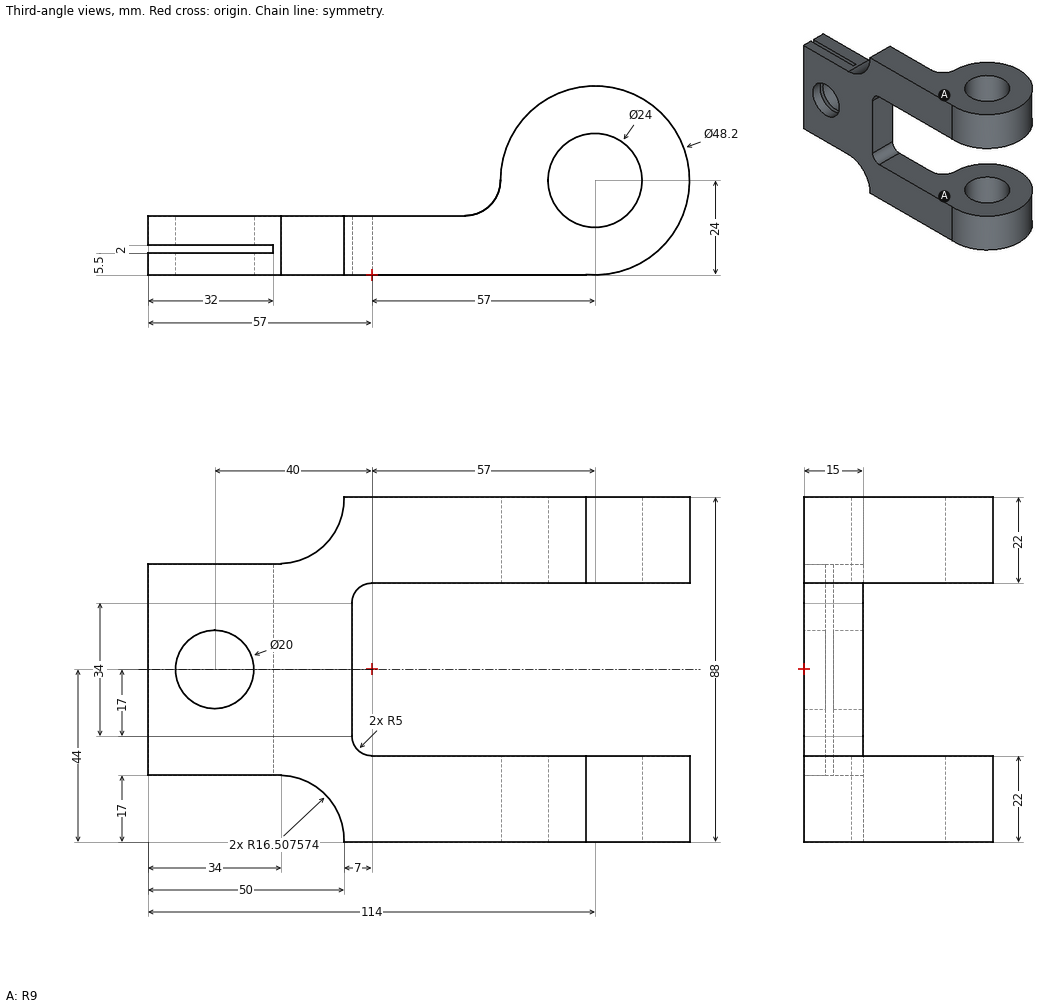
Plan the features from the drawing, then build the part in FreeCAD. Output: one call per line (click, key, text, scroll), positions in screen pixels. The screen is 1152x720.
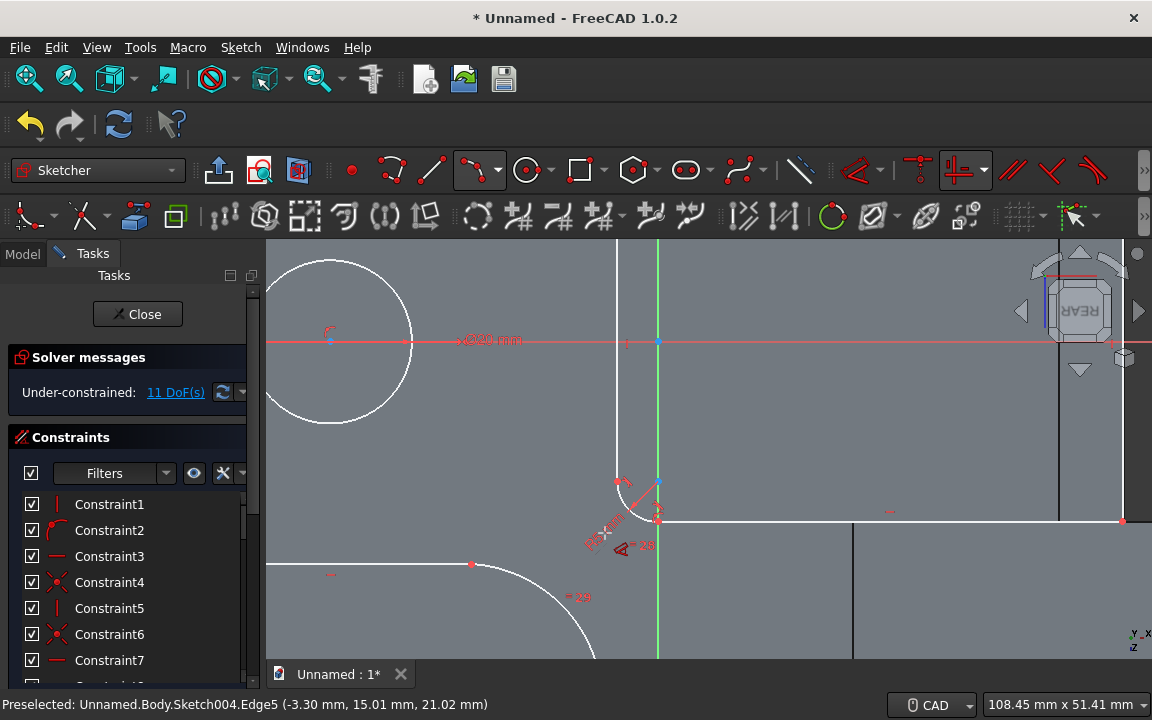
scroll(630, 511, down, 5)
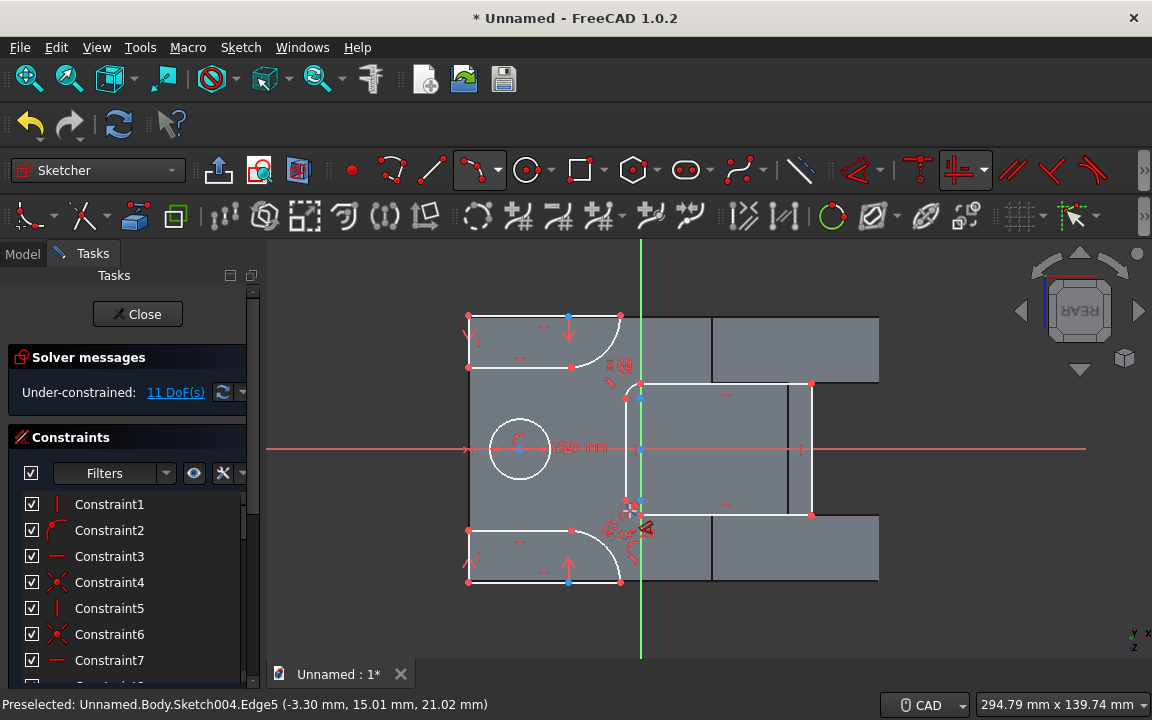
click(594, 361)
click(610, 389)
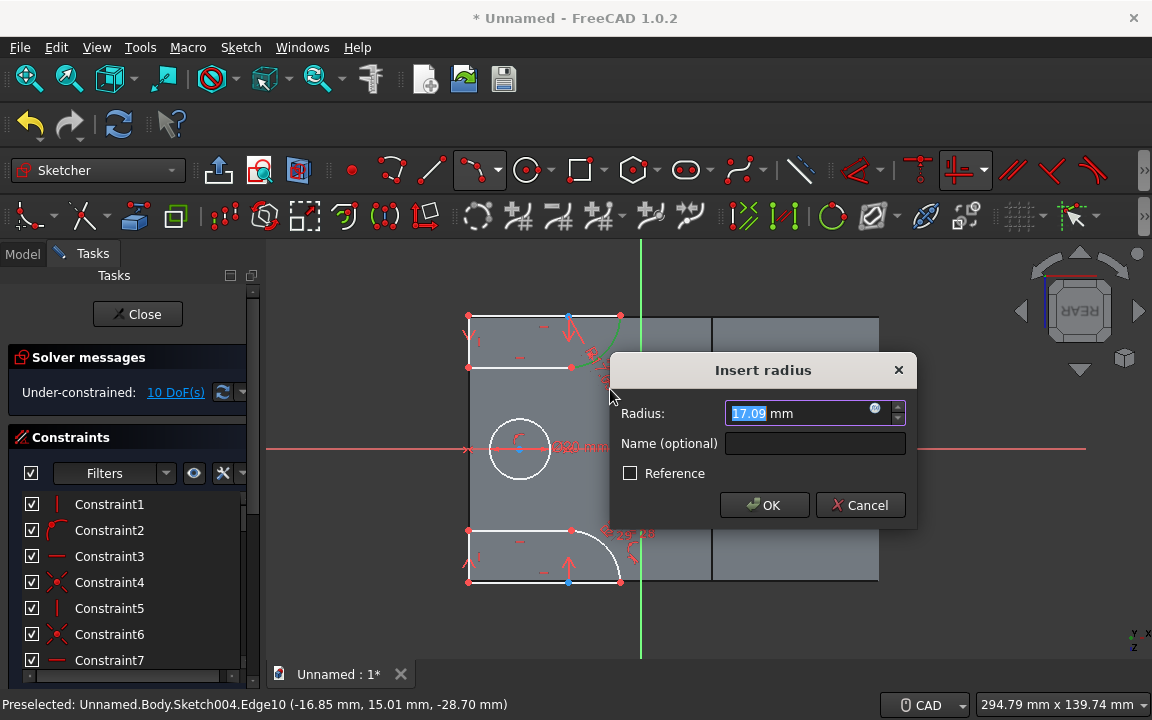
text(16.507574)
key(Return)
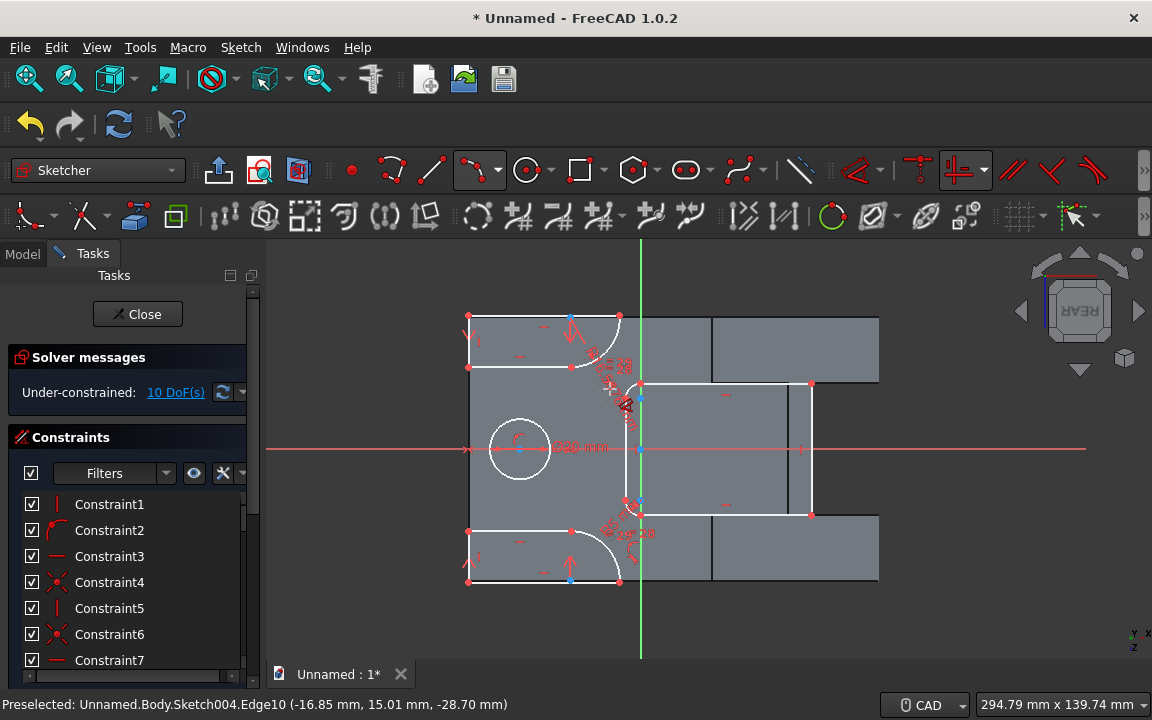
click(626, 429)
click(592, 426)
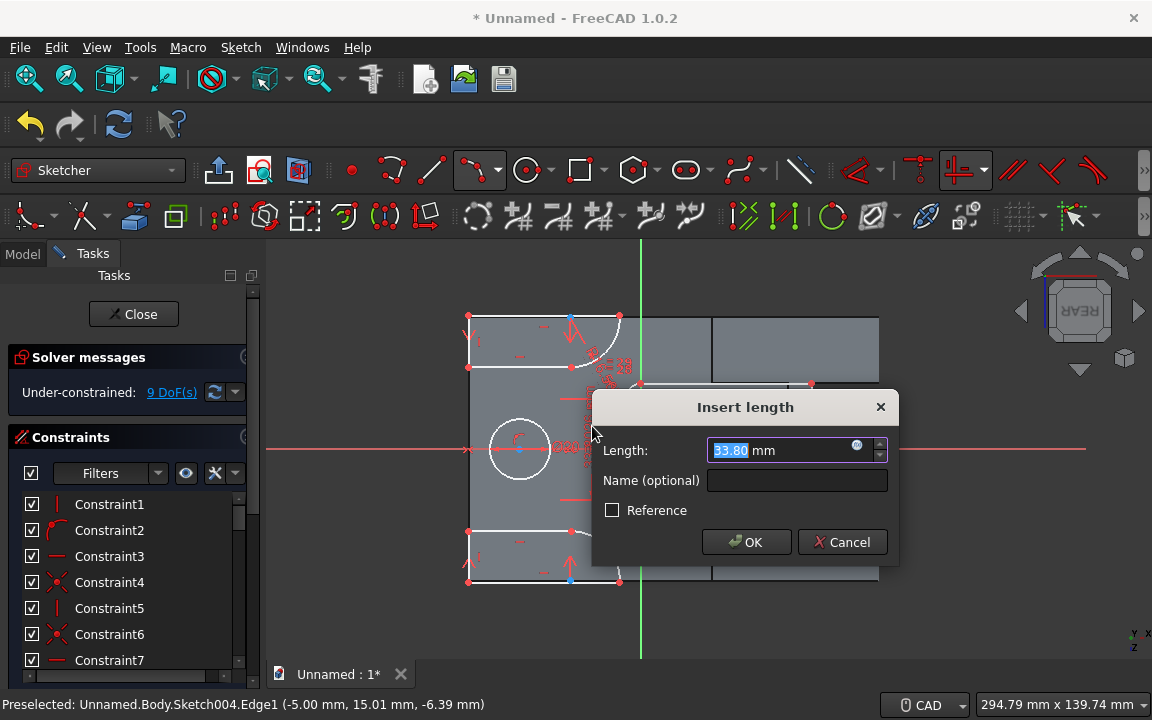
text(34)
key(Return)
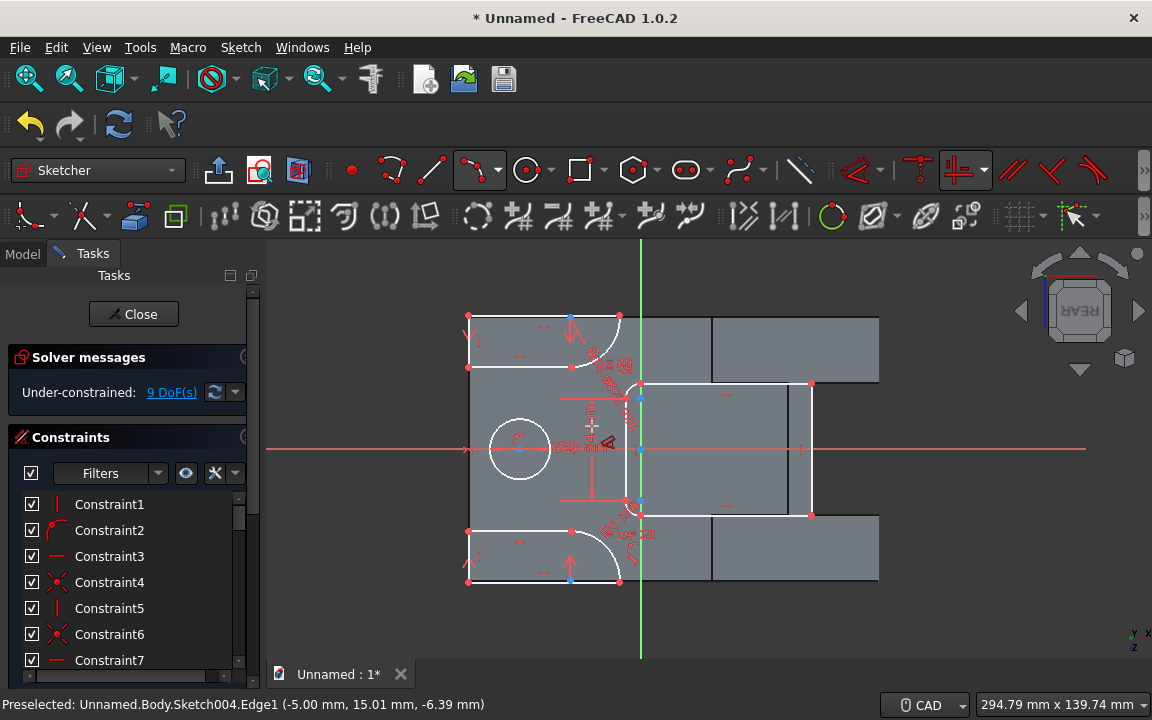
click(692, 516)
click(726, 550)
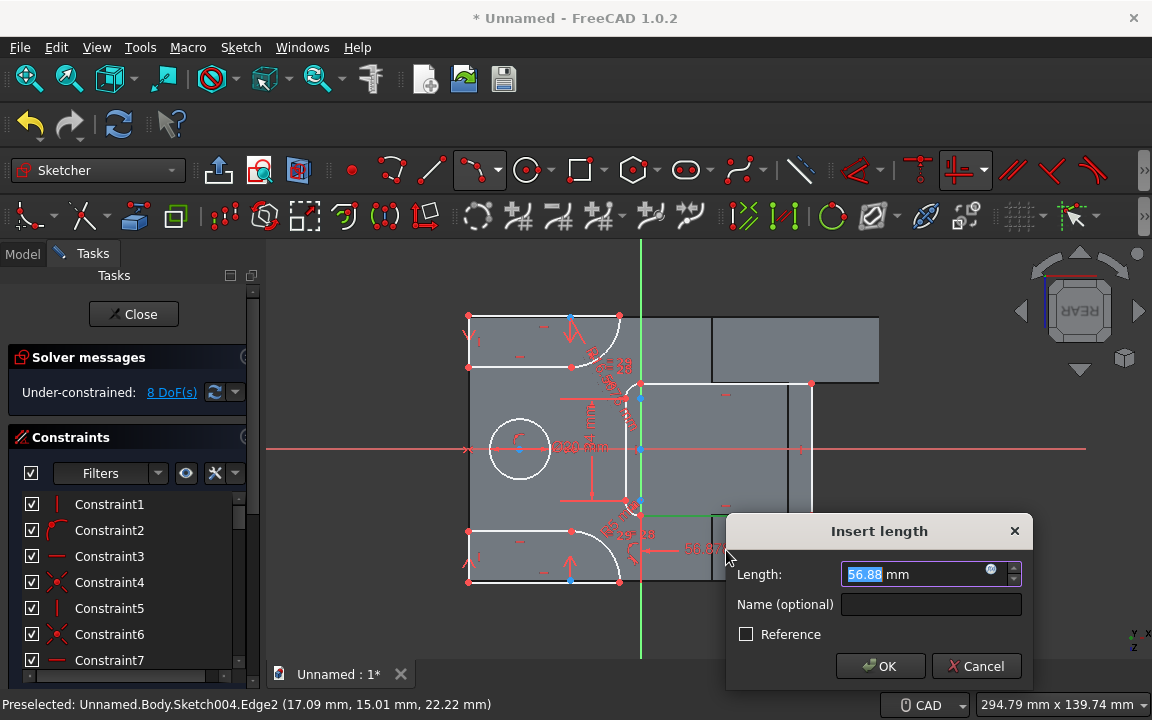
text(57)
key(Return)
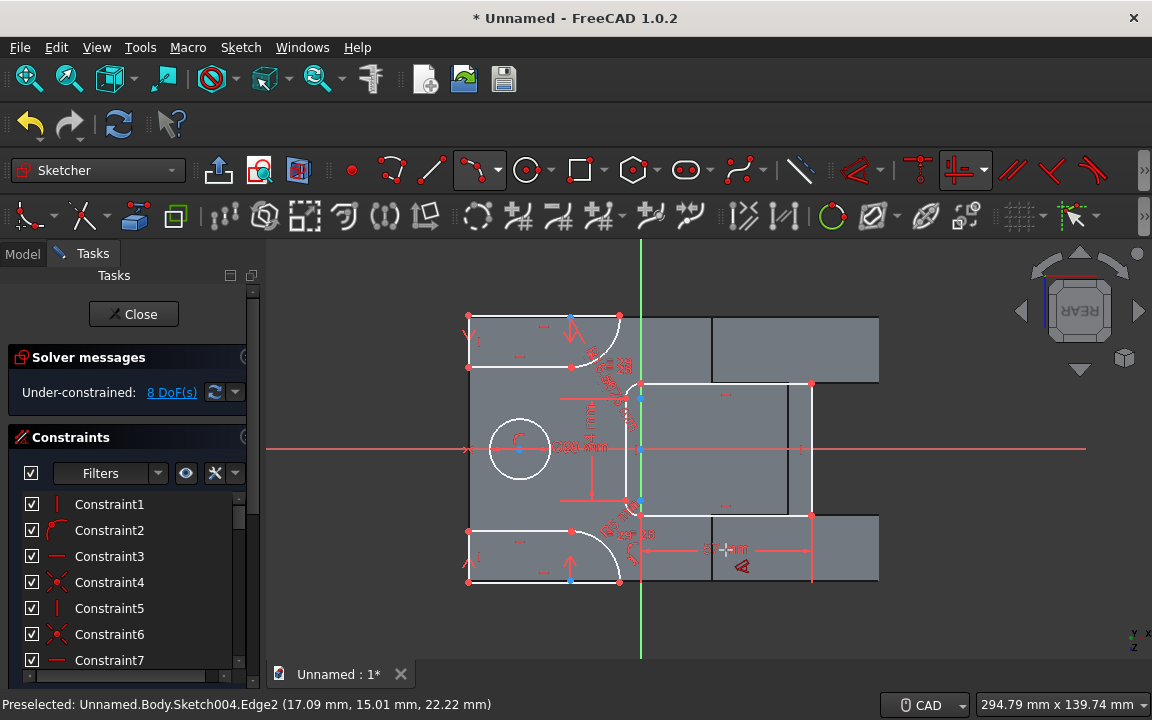
click(514, 316)
click(544, 282)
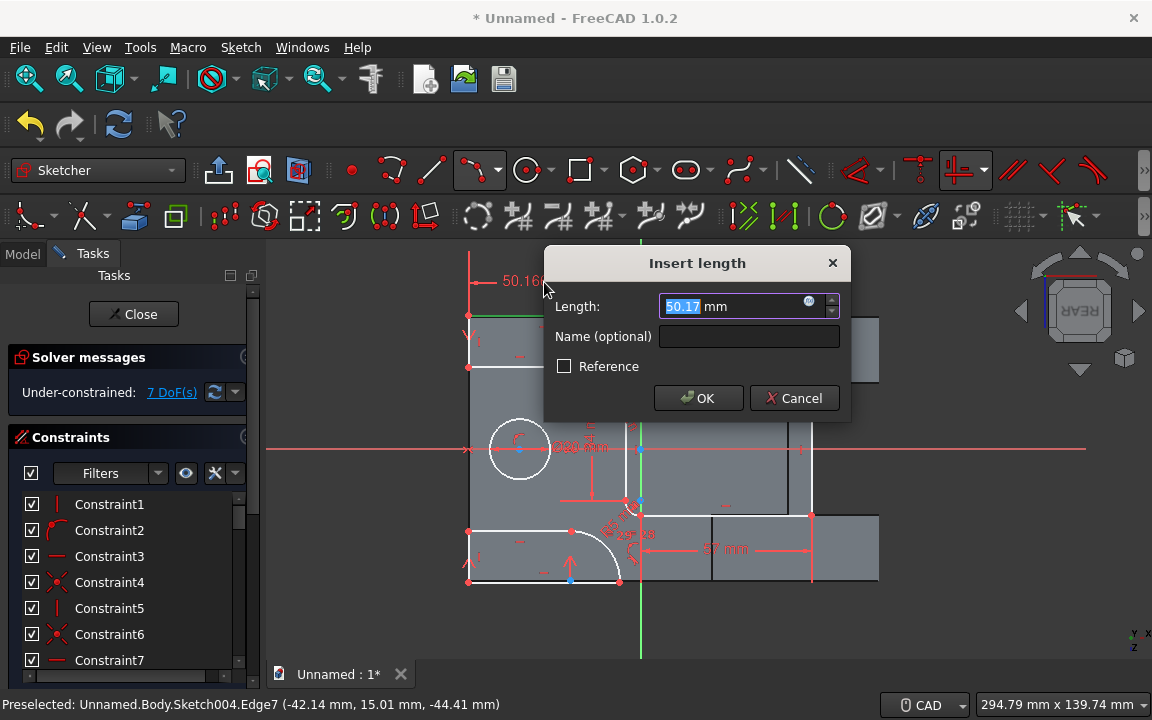
text(50)
key(Return)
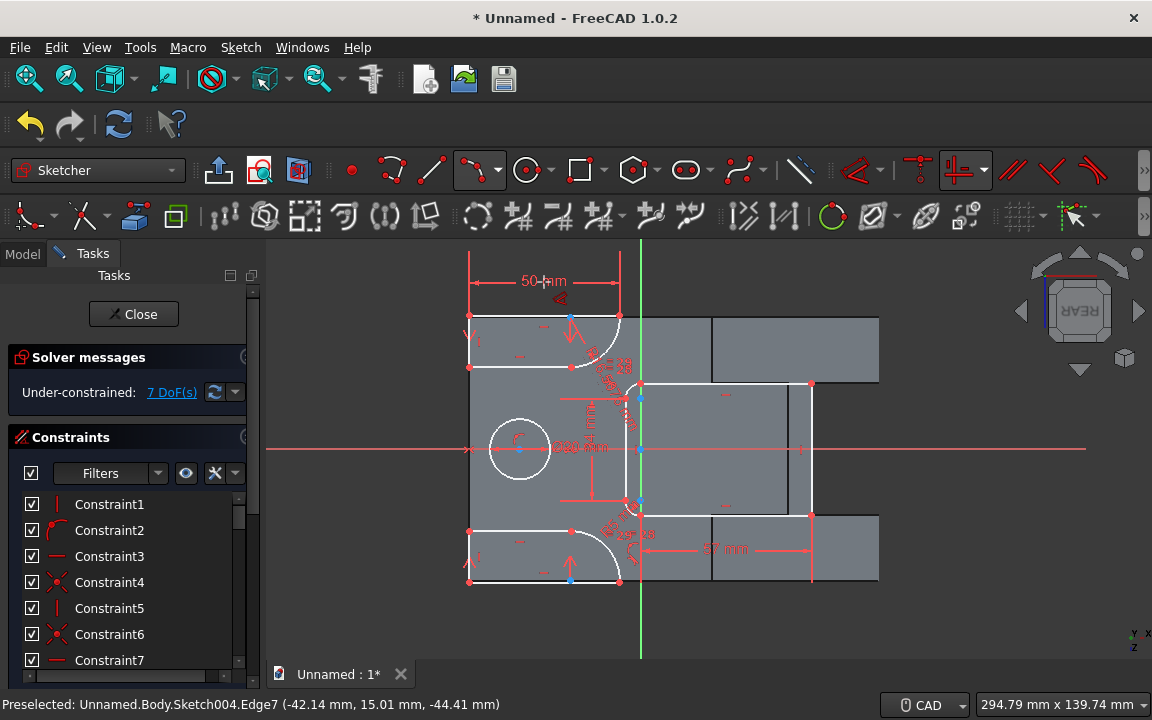
click(469, 331)
click(435, 342)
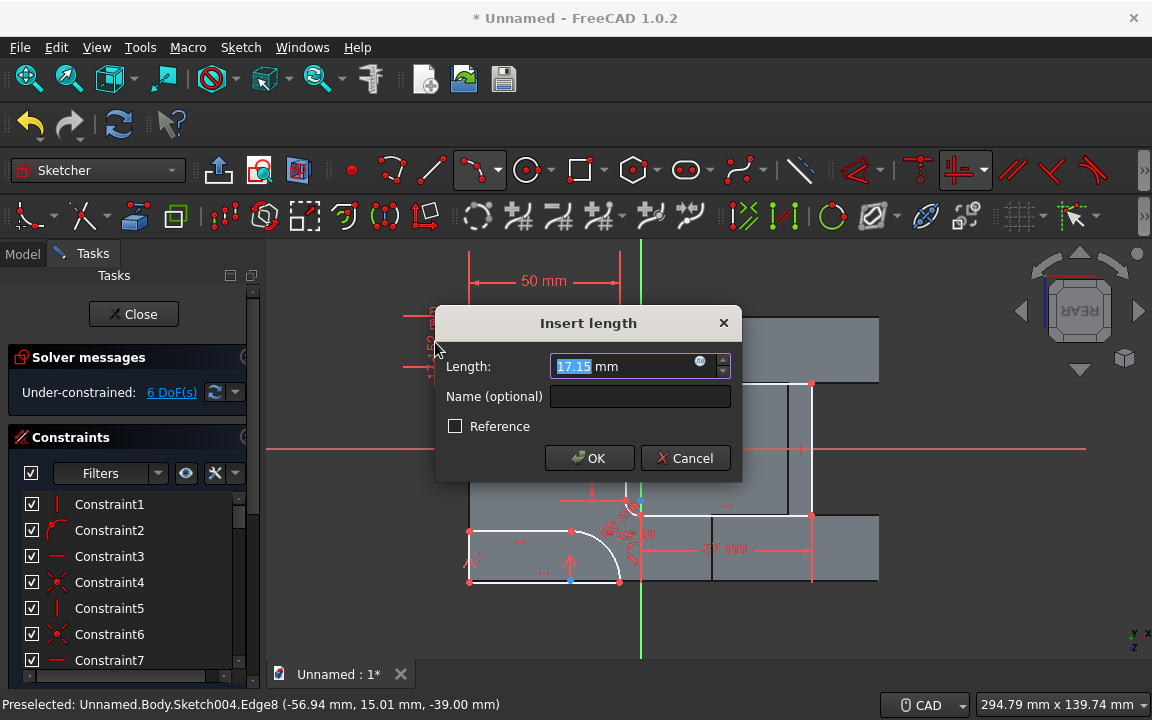
text(17)
key(Return)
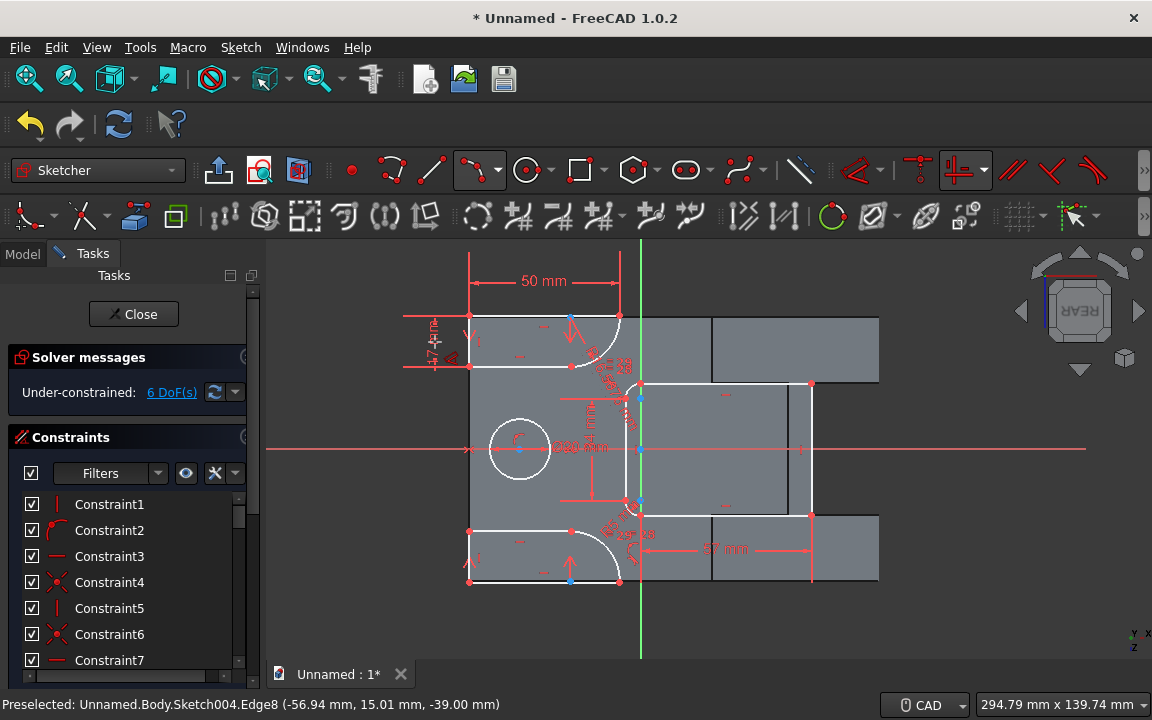
click(500, 367)
click(521, 333)